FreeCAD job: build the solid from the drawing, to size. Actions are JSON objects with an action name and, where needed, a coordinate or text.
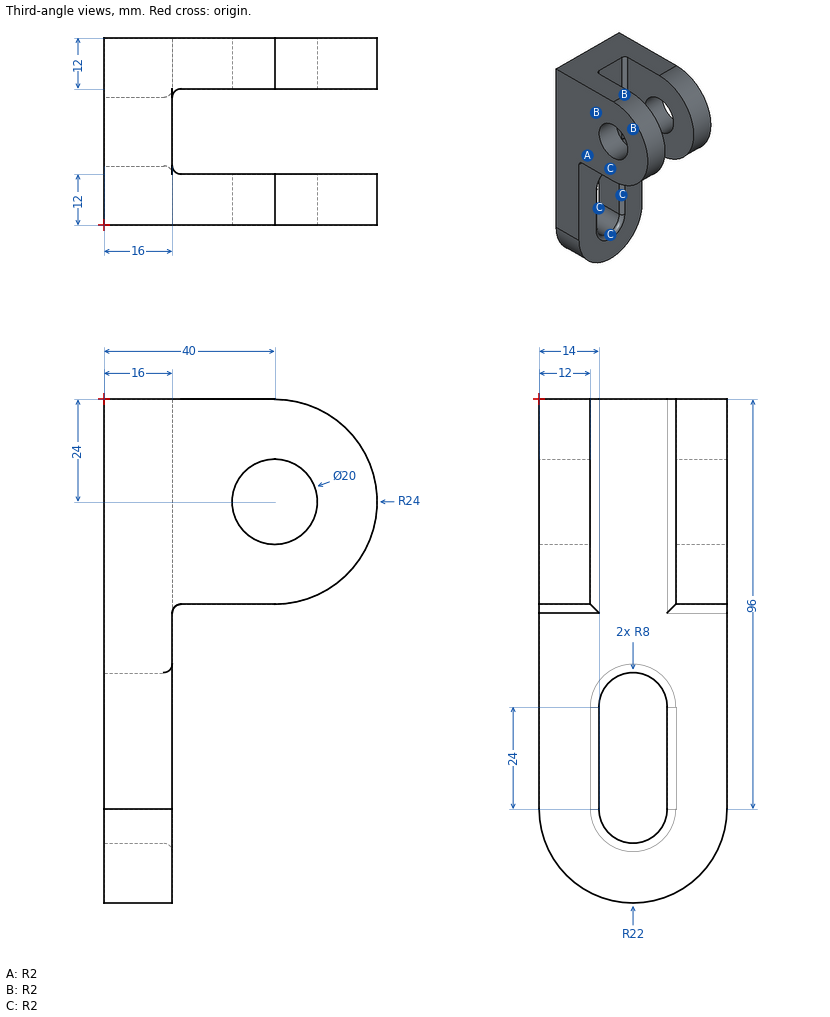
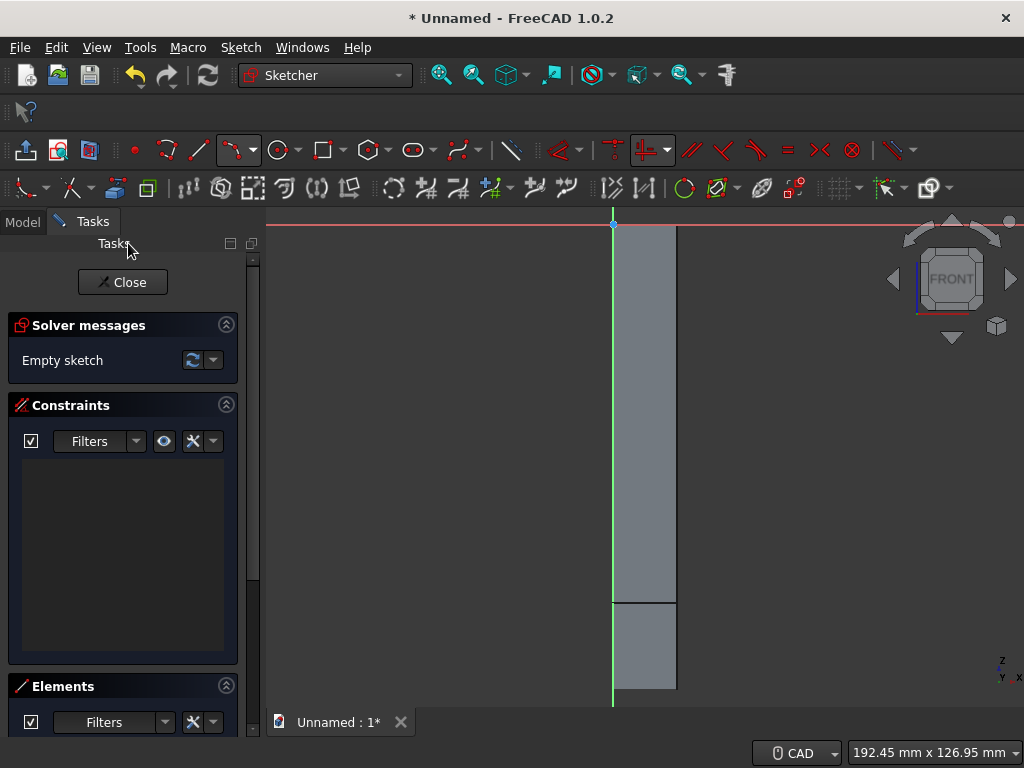
{"action": "scroll", "coordinate": [294, 679], "scroll_direction": "down", "scroll_amount": 1}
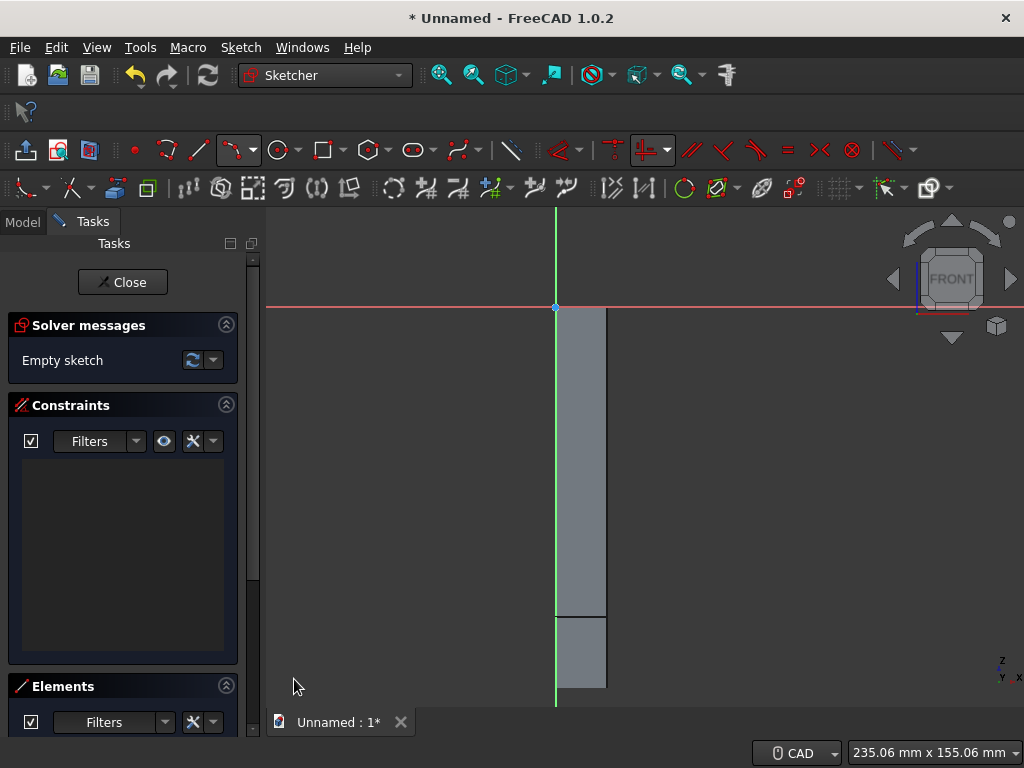
{"action": "scroll", "coordinate": [759, 296], "scroll_direction": "up", "scroll_amount": 3}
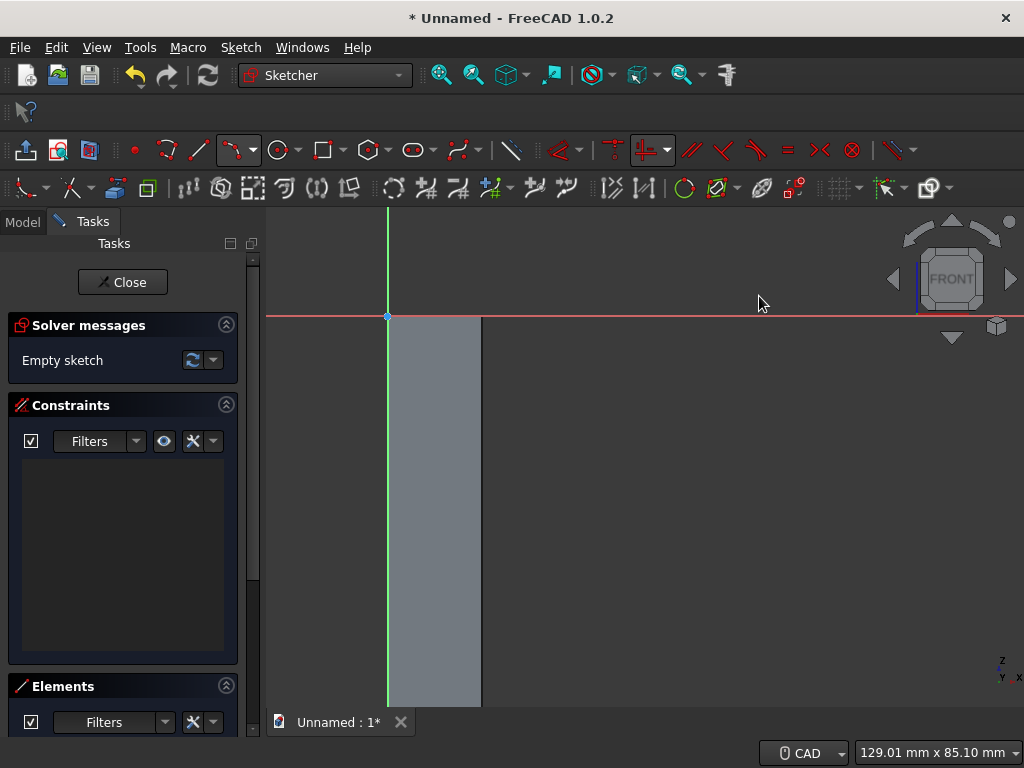
{"action": "left_click", "coordinate": [168, 150]}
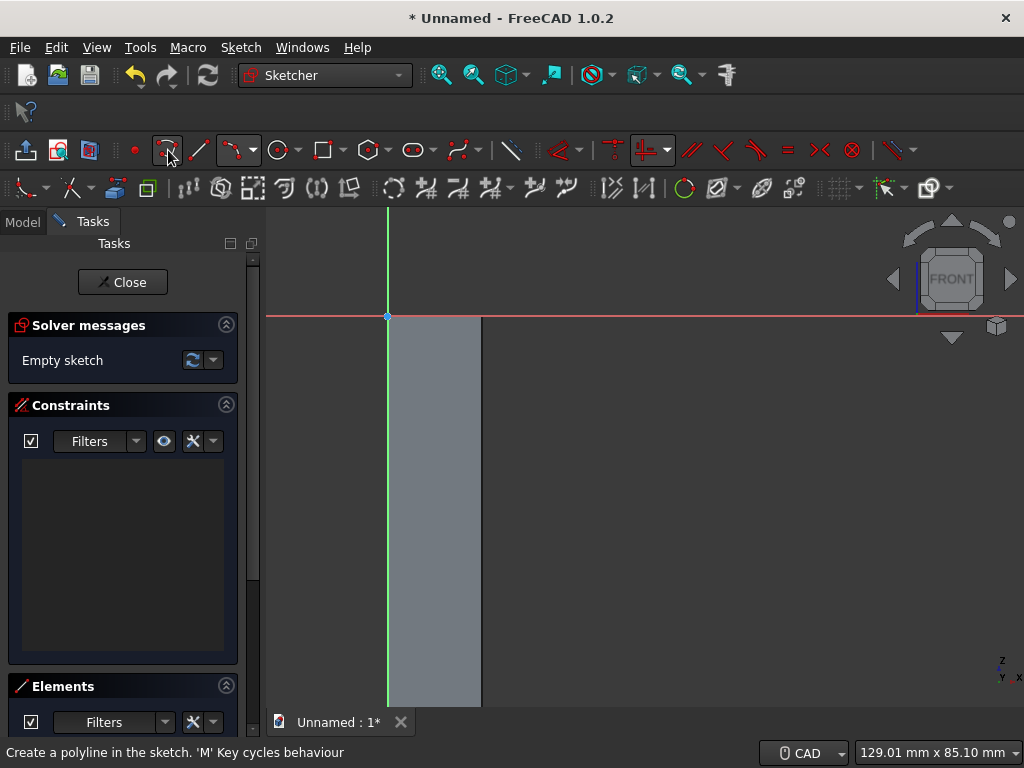
{"action": "left_click", "coordinate": [623, 316]}
{"action": "left_click", "coordinate": [388, 316]}
{"action": "left_click", "coordinate": [397, 598]}
{"action": "left_click", "coordinate": [623, 598]}
{"action": "right_click", "coordinate": [623, 598]}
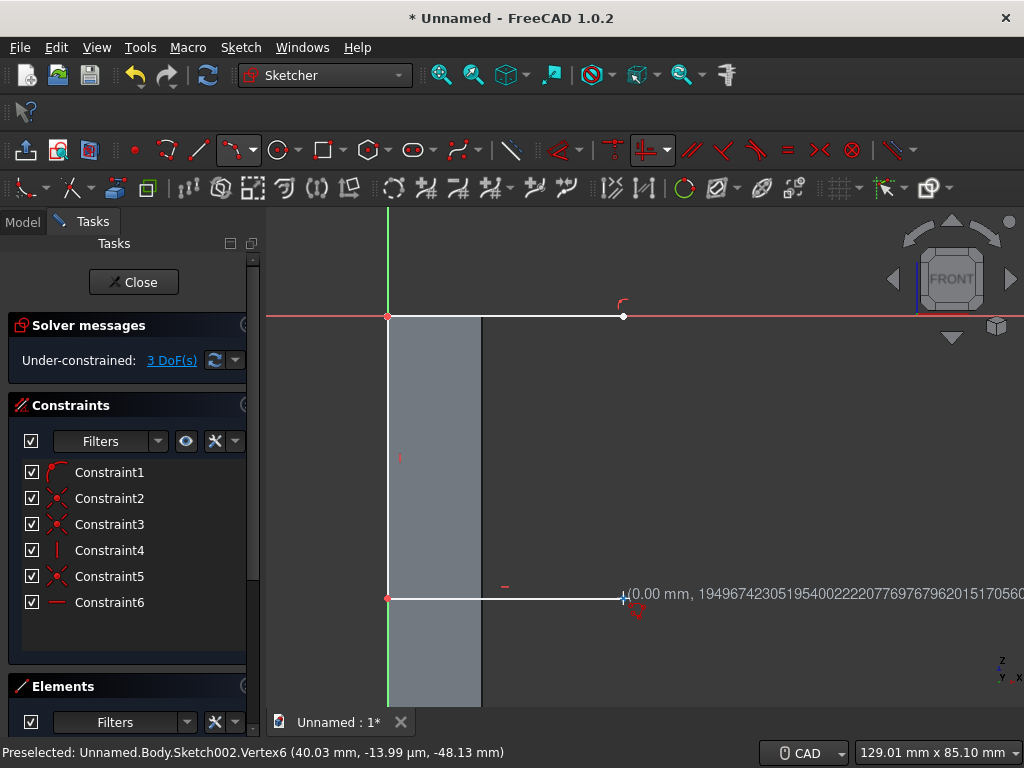
{"action": "left_click", "coordinate": [232, 150]}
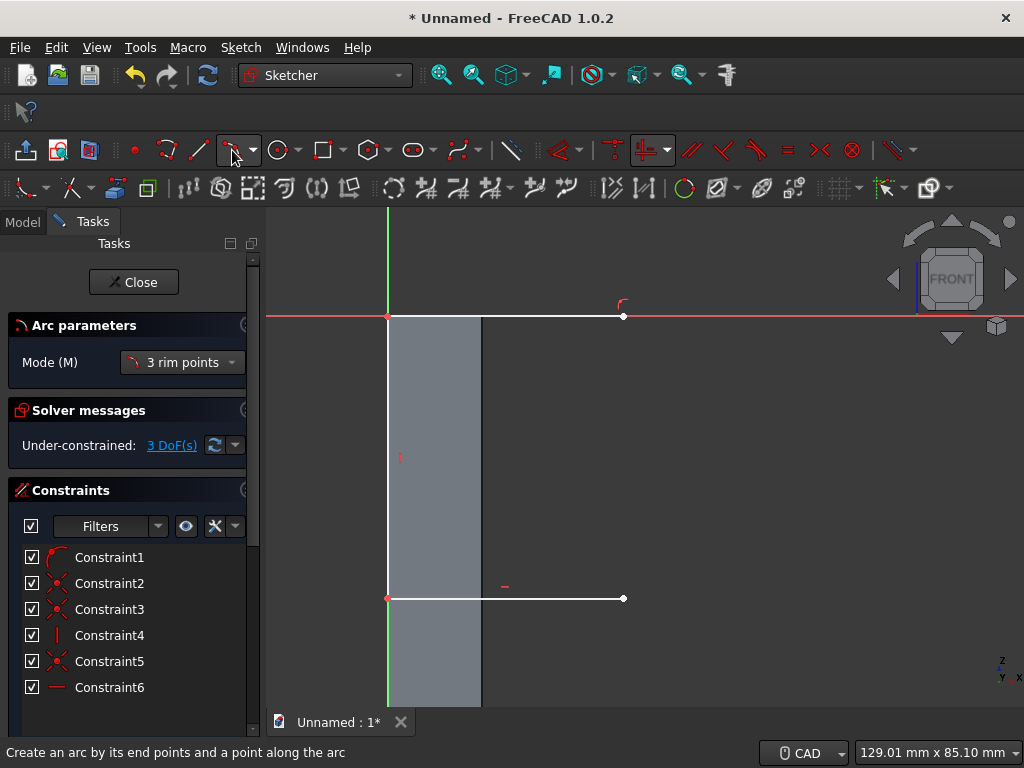
{"action": "left_click", "coordinate": [623, 599]}
{"action": "left_click", "coordinate": [623, 316]}
{"action": "left_click", "coordinate": [764, 457]}
{"action": "key", "text": "Escape"}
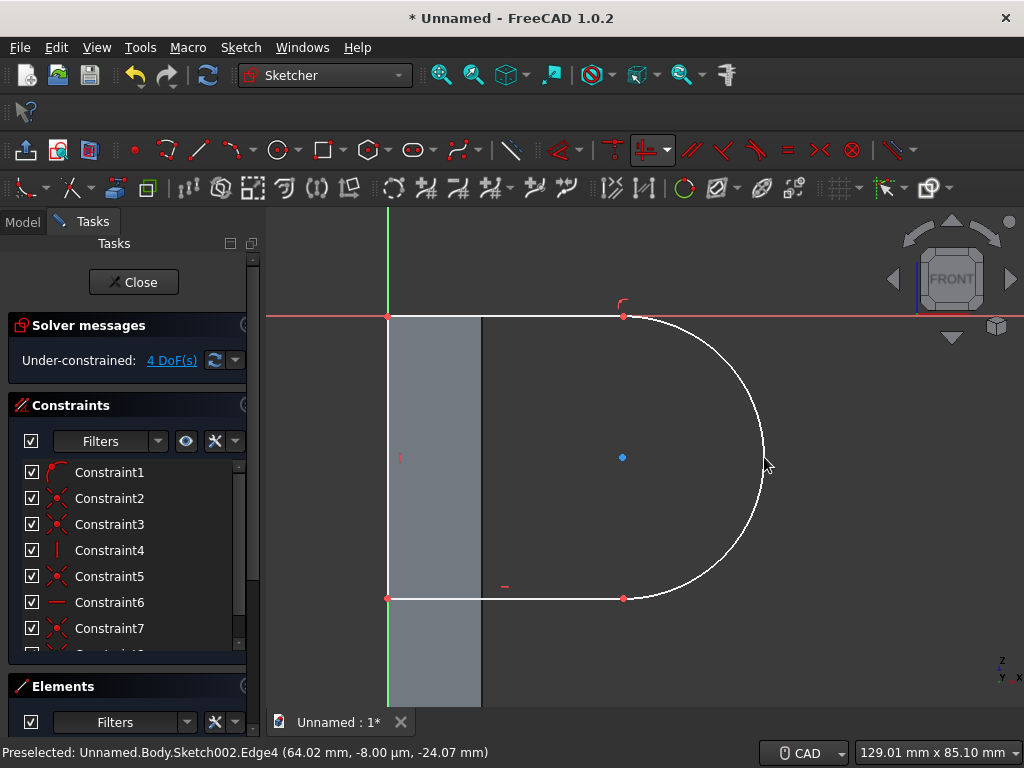
{"action": "left_click", "coordinate": [552, 316]}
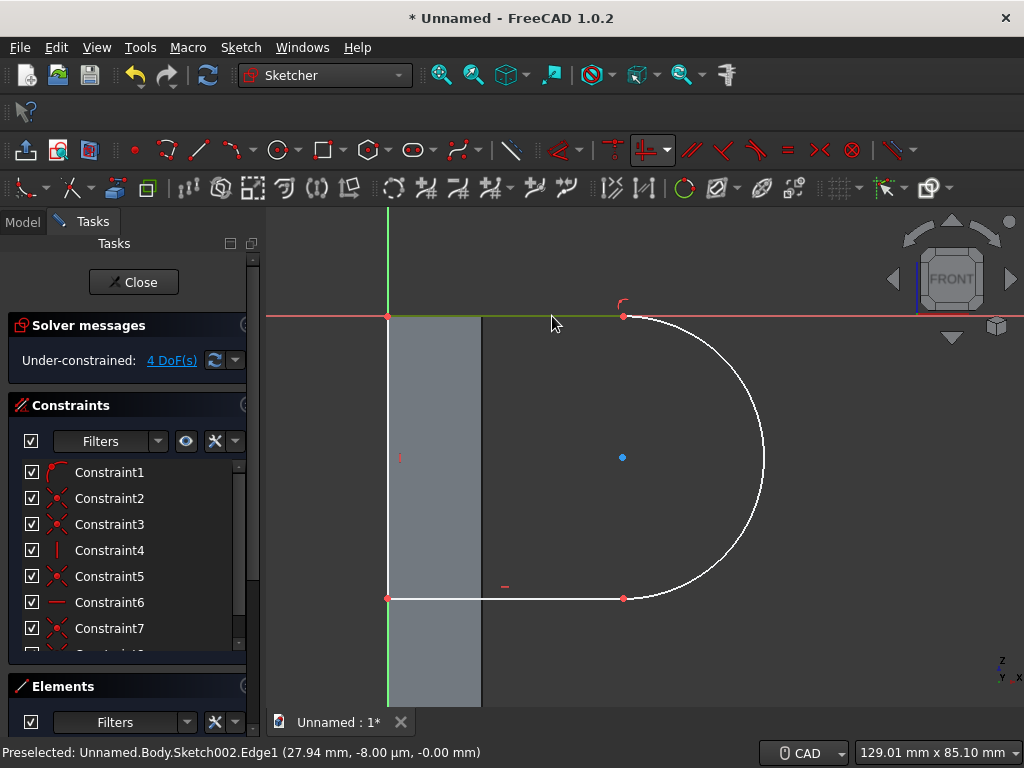
{"action": "left_click", "coordinate": [737, 541]}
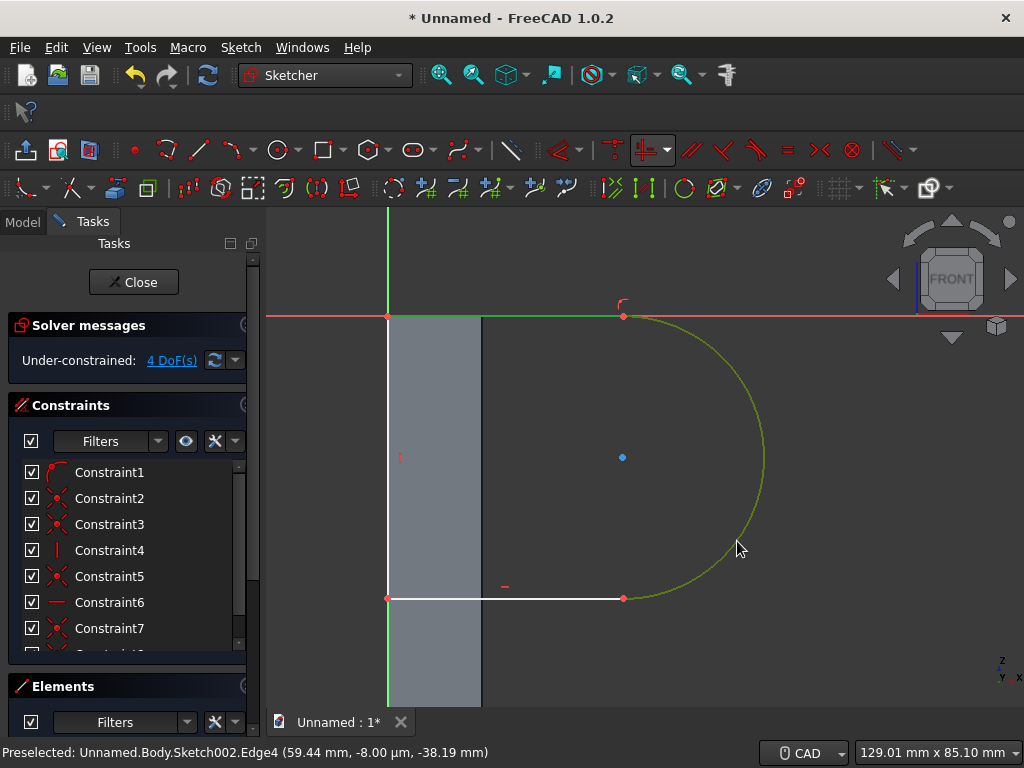
{"action": "left_click", "coordinate": [756, 150]}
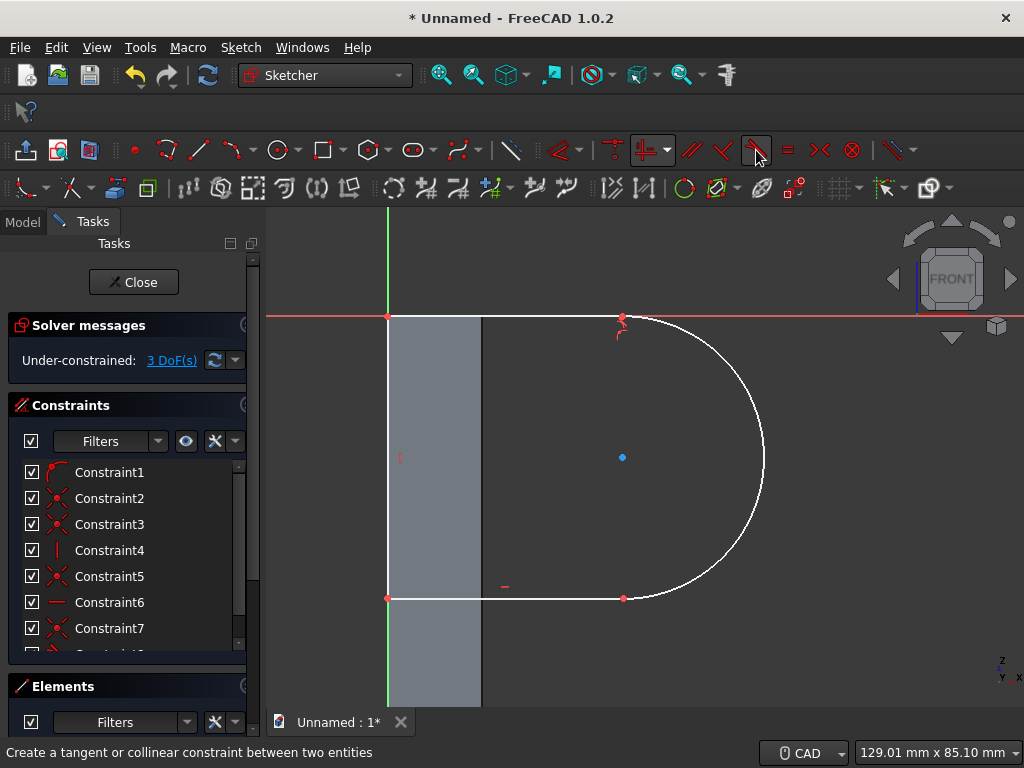
{"action": "left_click", "coordinate": [458, 599]}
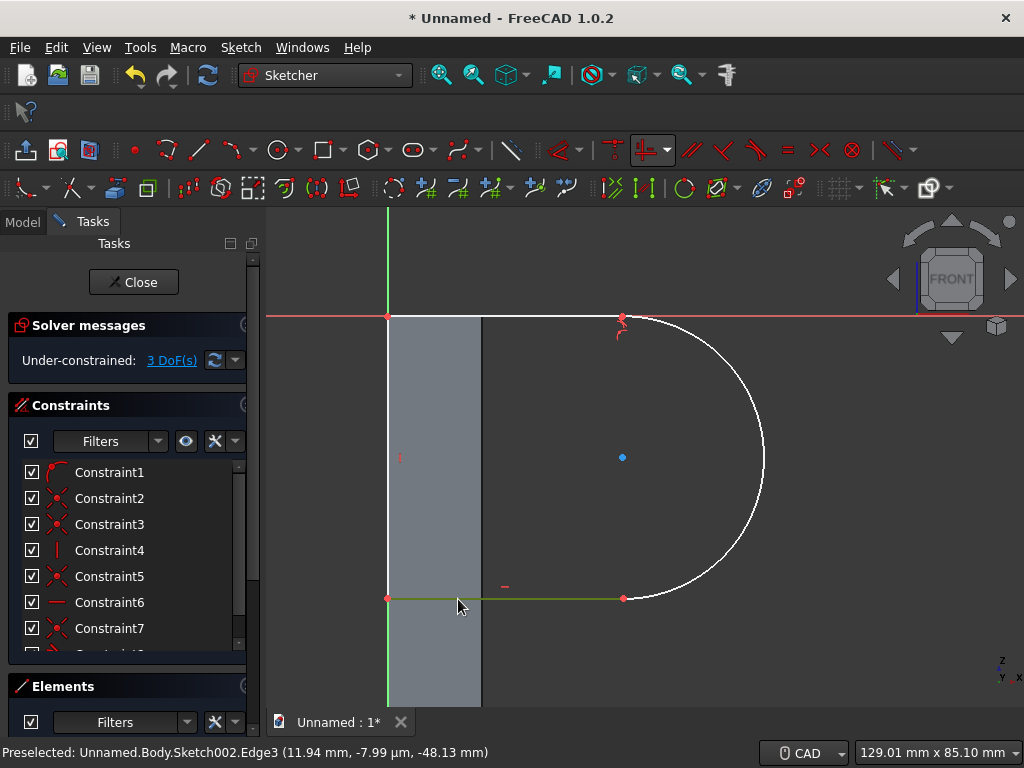
{"action": "left_click", "coordinate": [737, 540]}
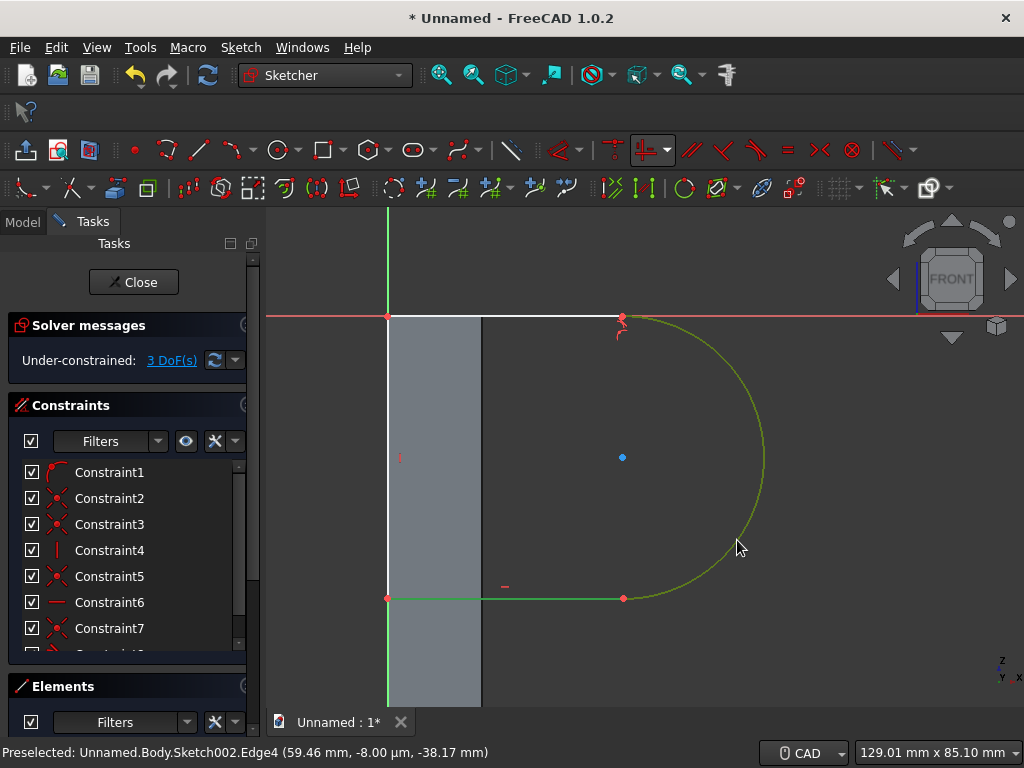
{"action": "left_click", "coordinate": [756, 150]}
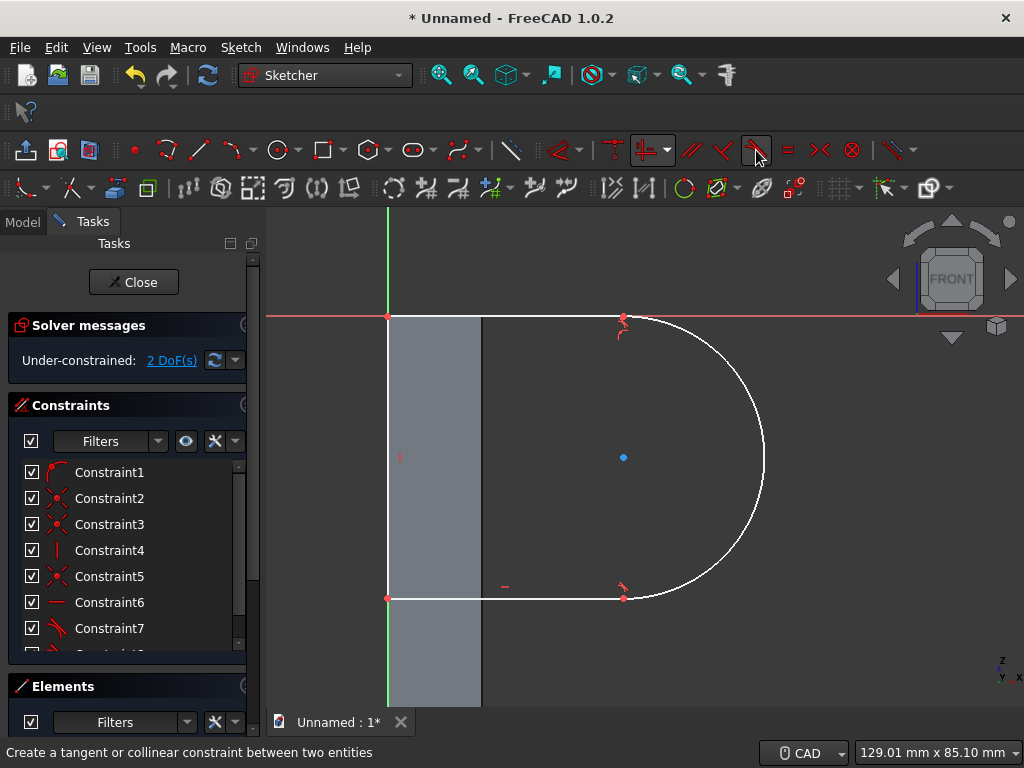
{"action": "left_click", "coordinate": [558, 150]}